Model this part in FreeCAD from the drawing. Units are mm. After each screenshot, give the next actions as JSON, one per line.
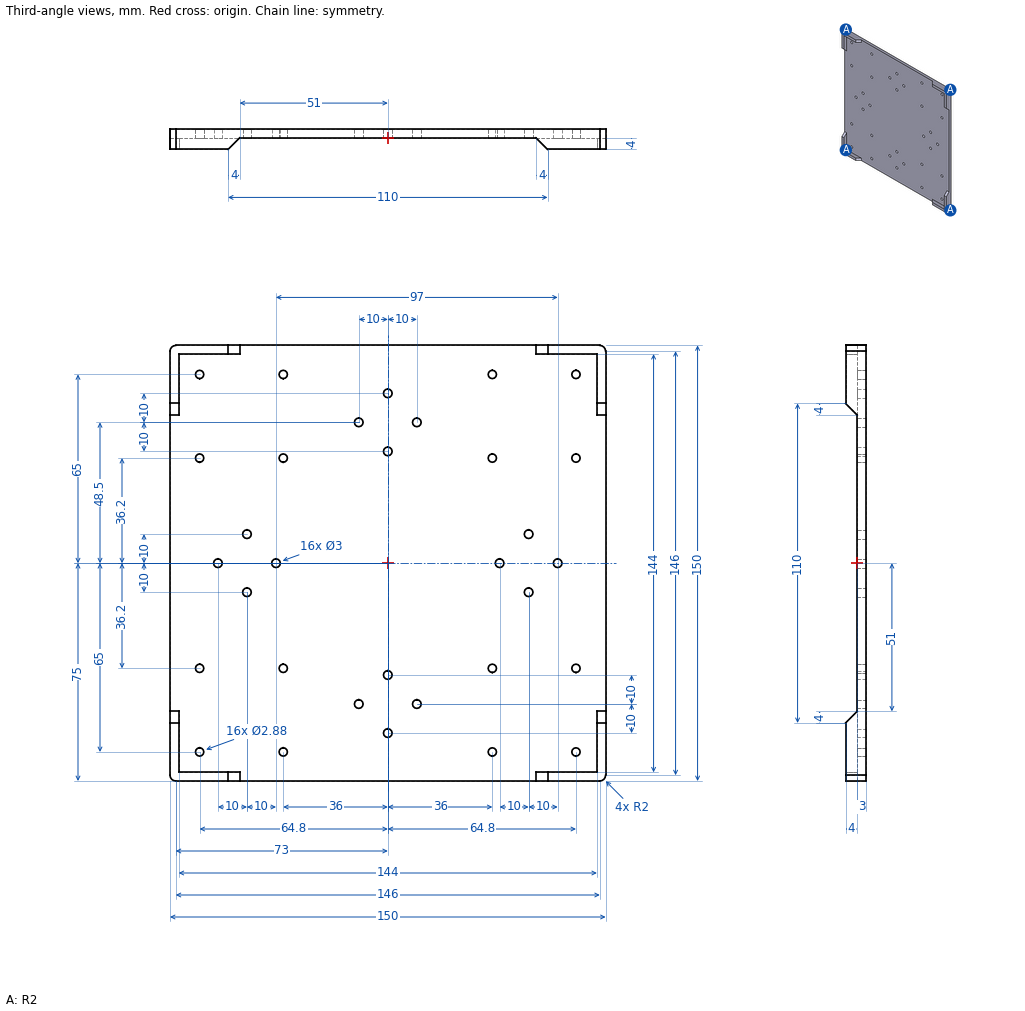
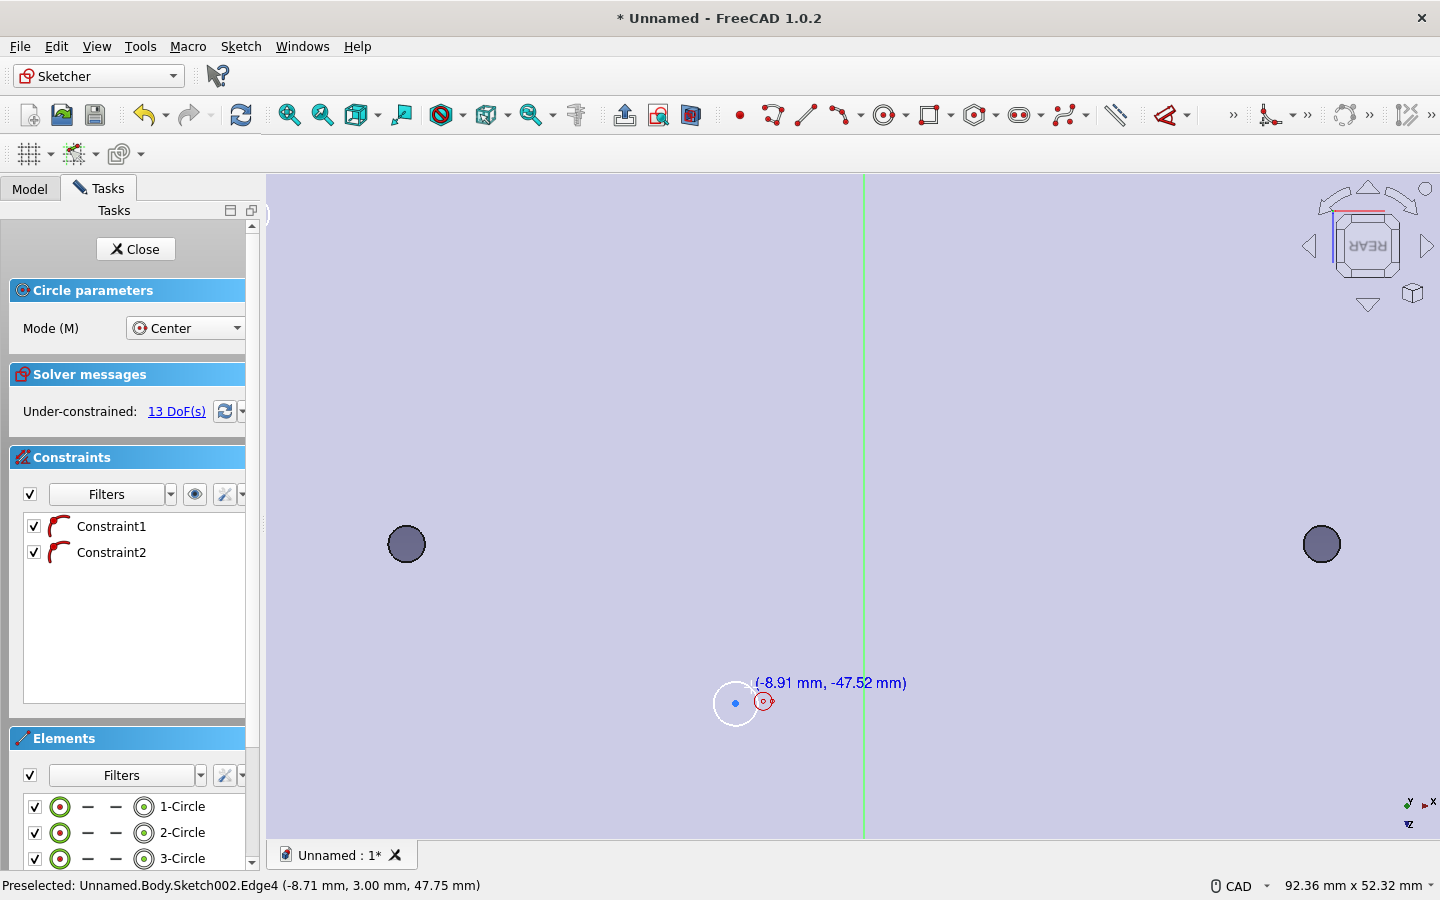
{"action": "scroll", "coordinate": [750, 689], "scroll_direction": "down", "scroll_amount": 6}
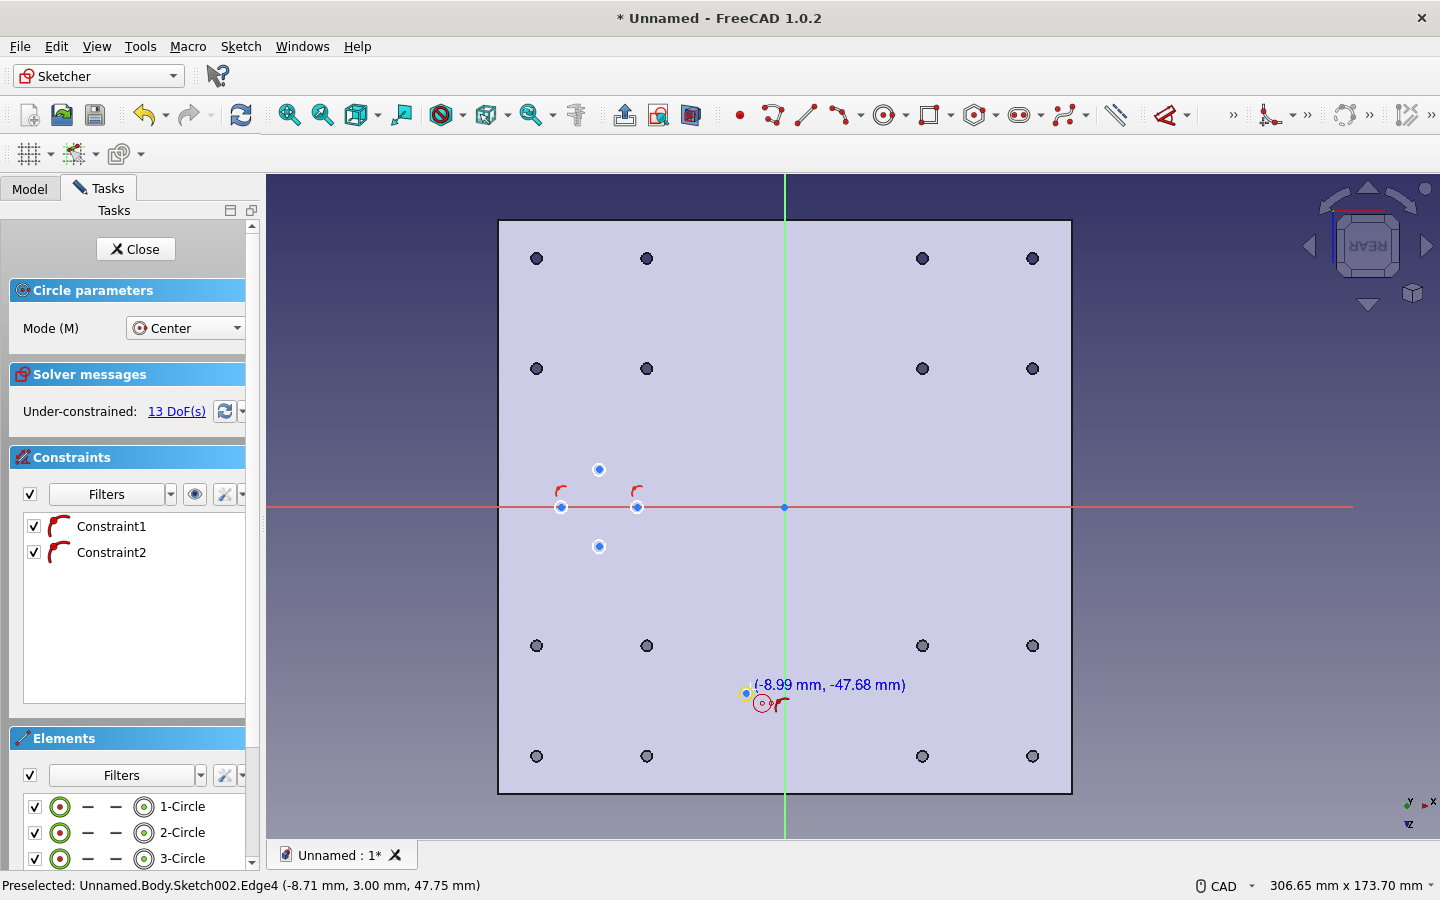
{"action": "scroll", "coordinate": [785, 731], "scroll_direction": "up", "scroll_amount": 7}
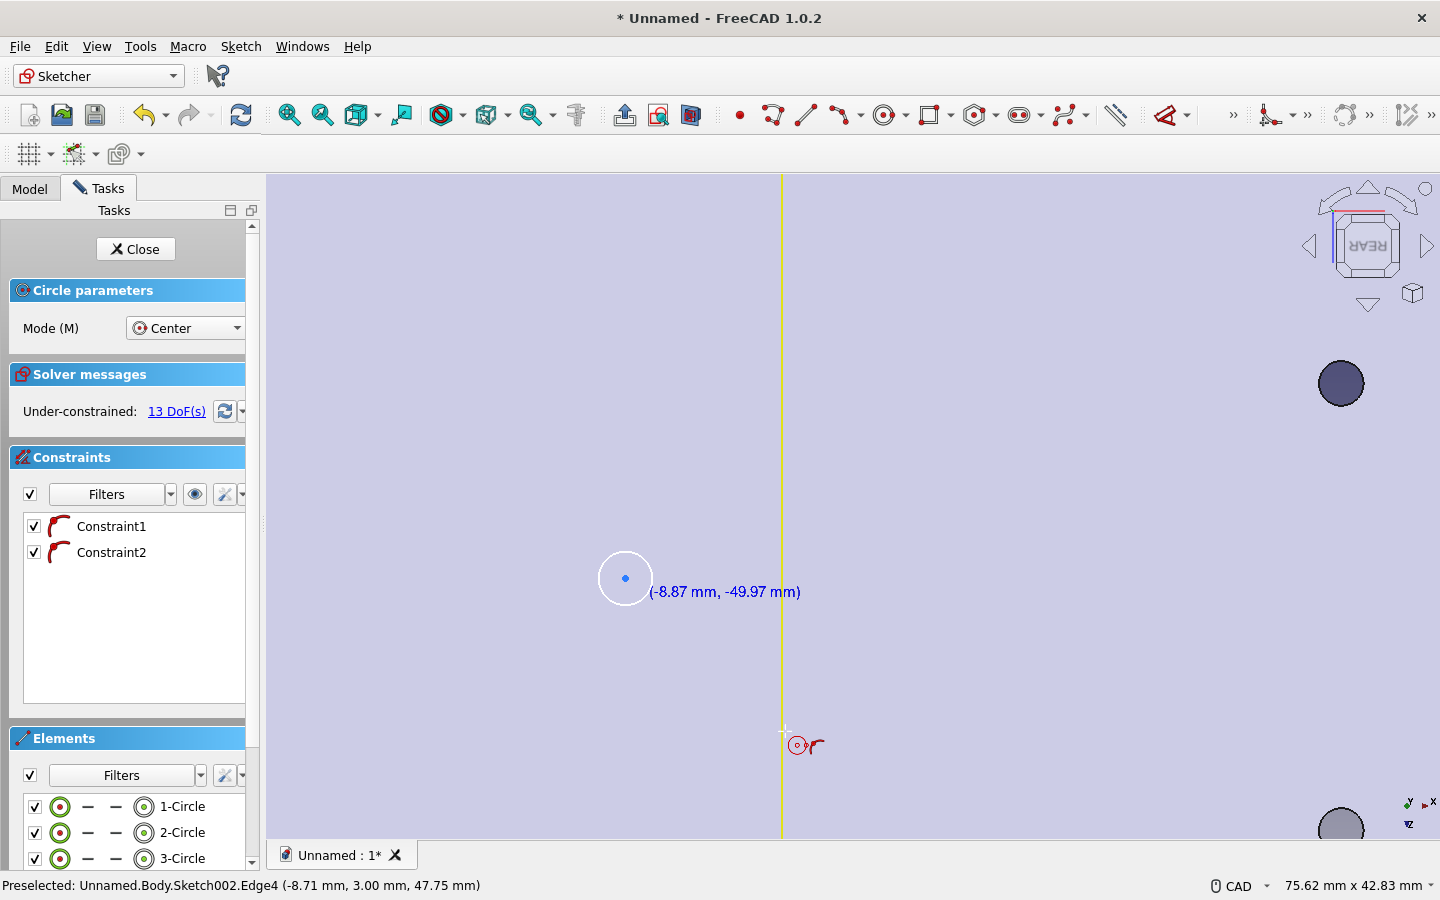
{"action": "scroll", "coordinate": [785, 731], "scroll_direction": "down", "scroll_amount": 7}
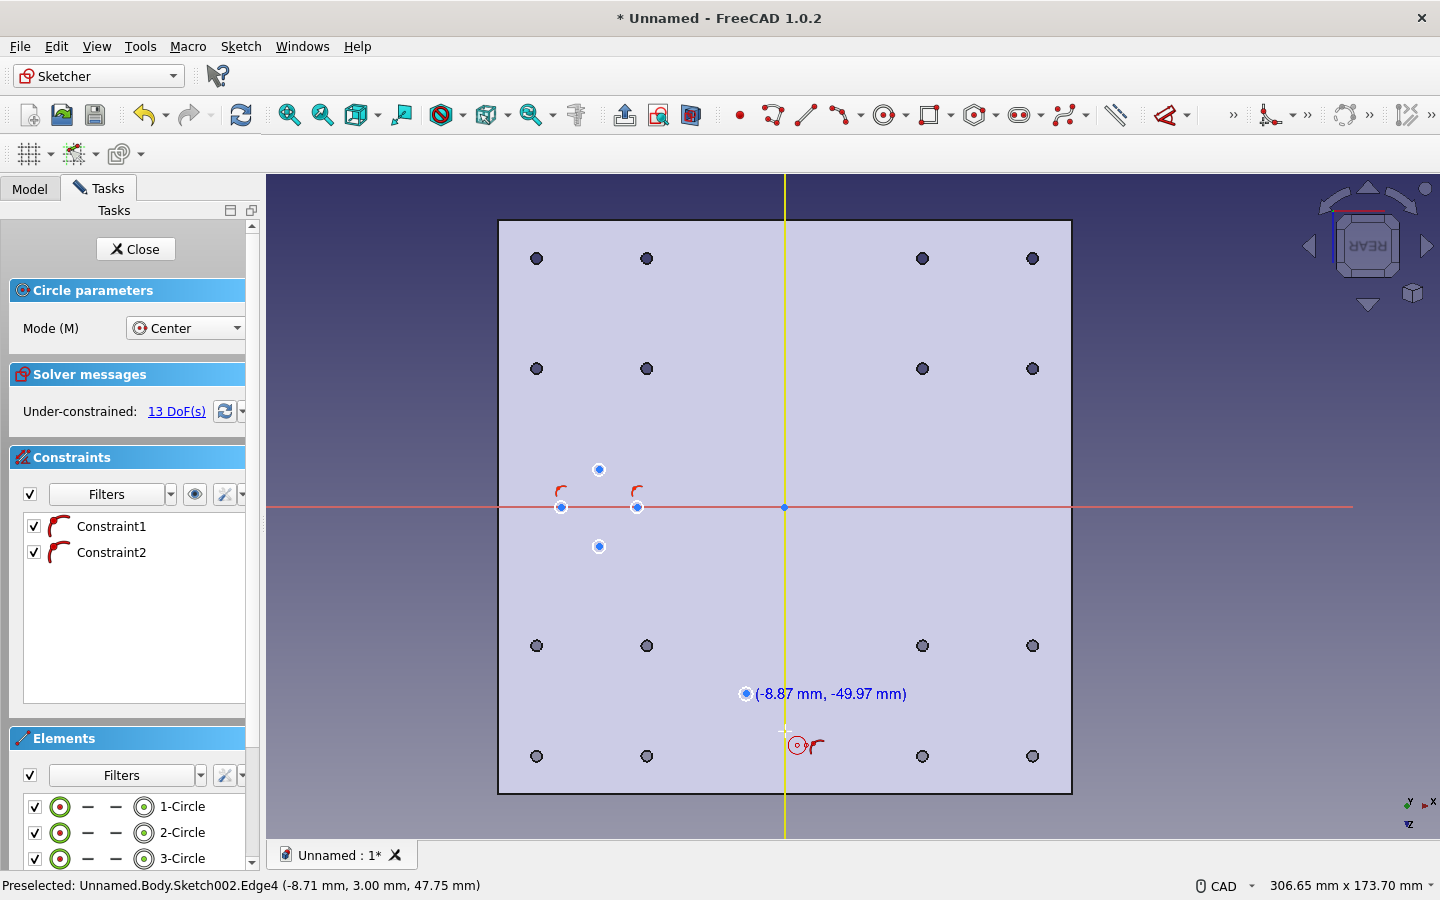
{"action": "left_click", "coordinate": [785, 731]}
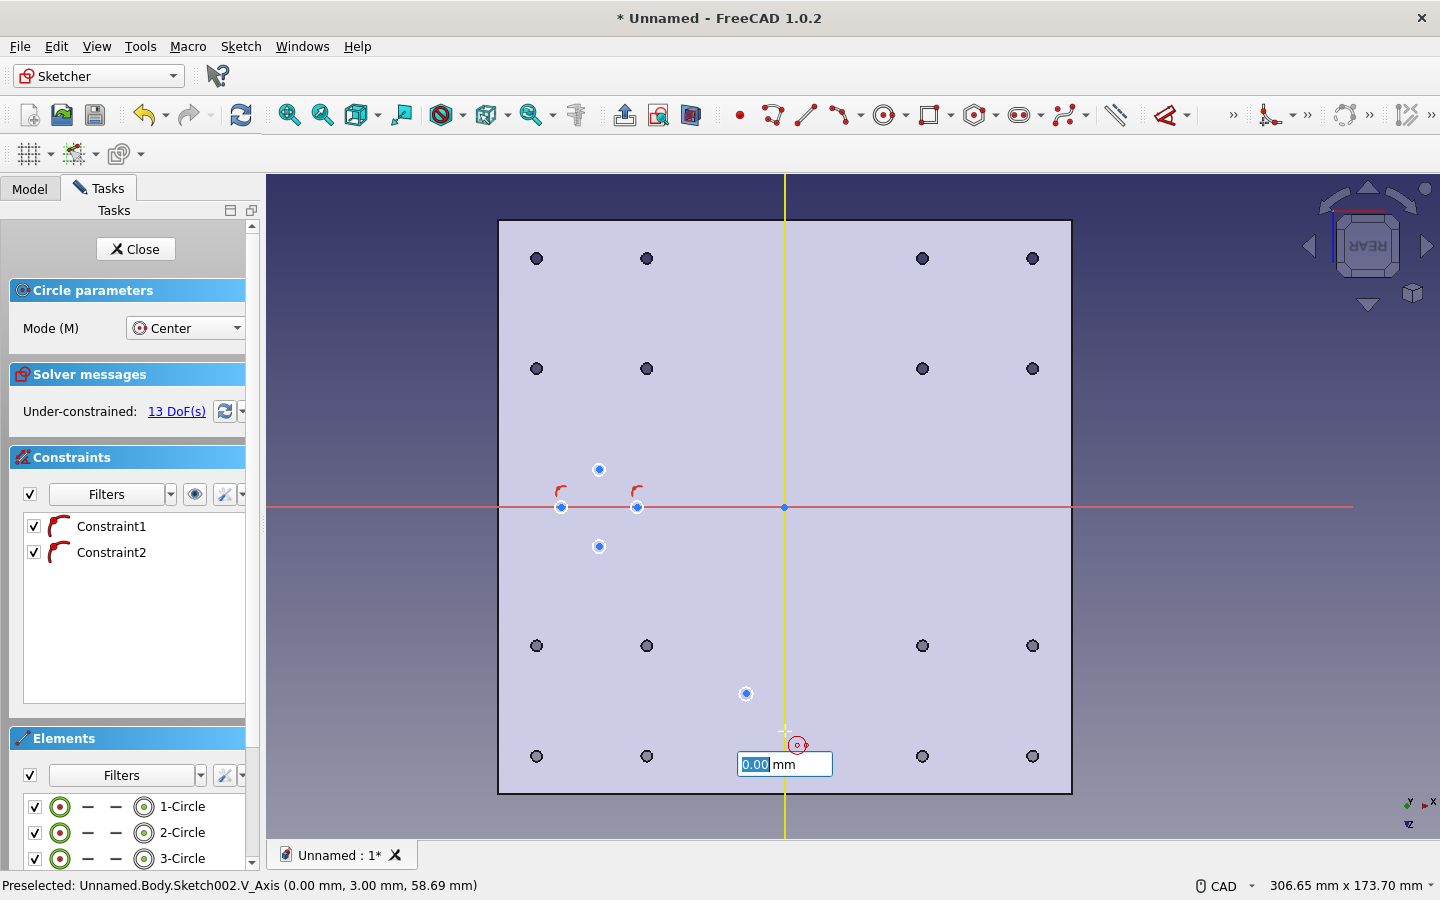
{"action": "scroll", "coordinate": [790, 729], "scroll_direction": "up", "scroll_amount": 6}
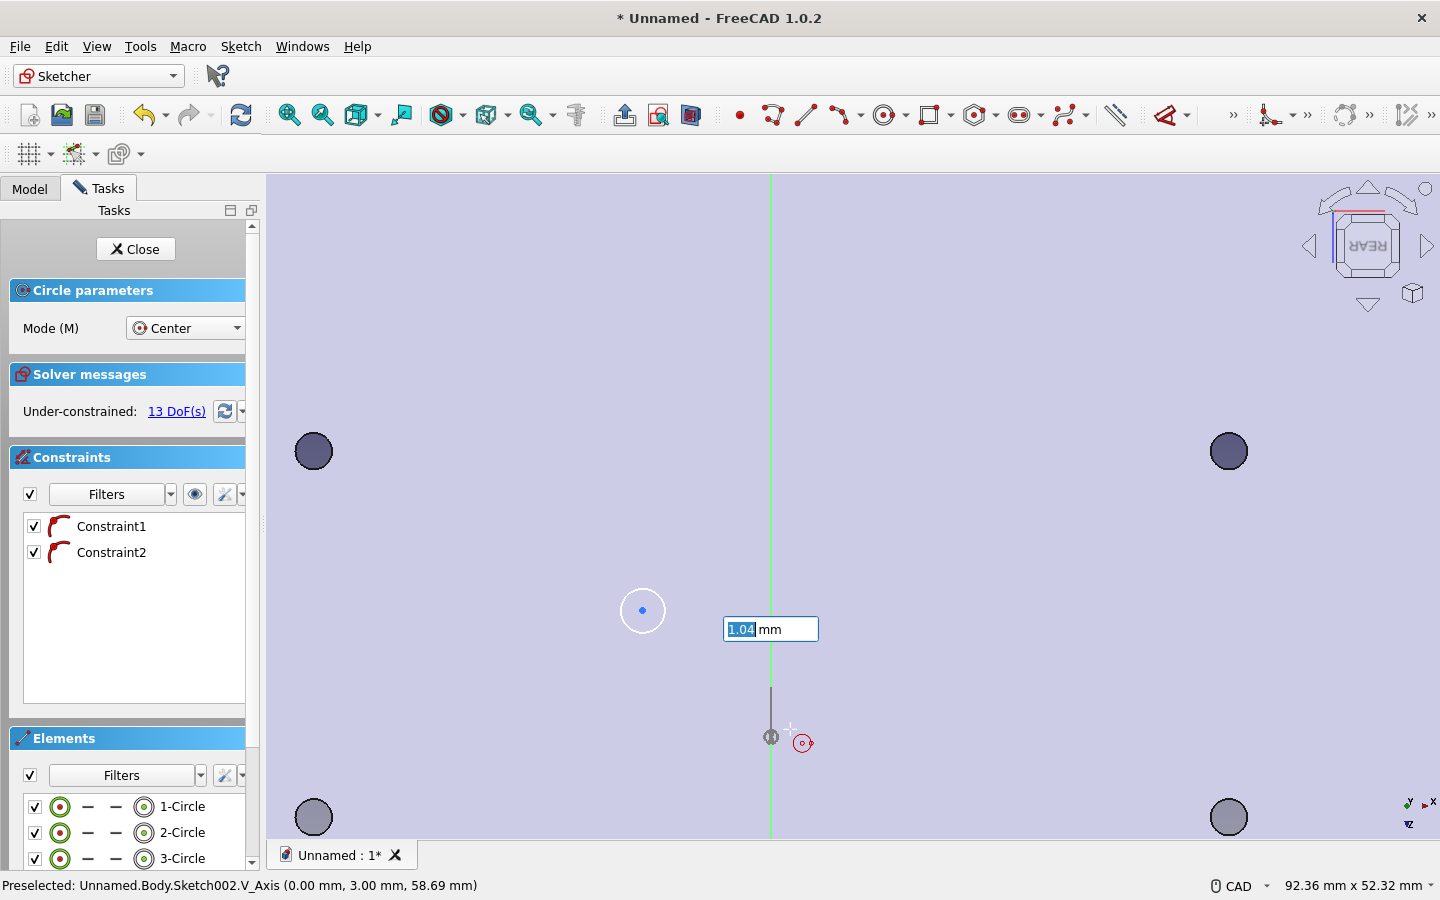
{"action": "left_click", "coordinate": [789, 728]}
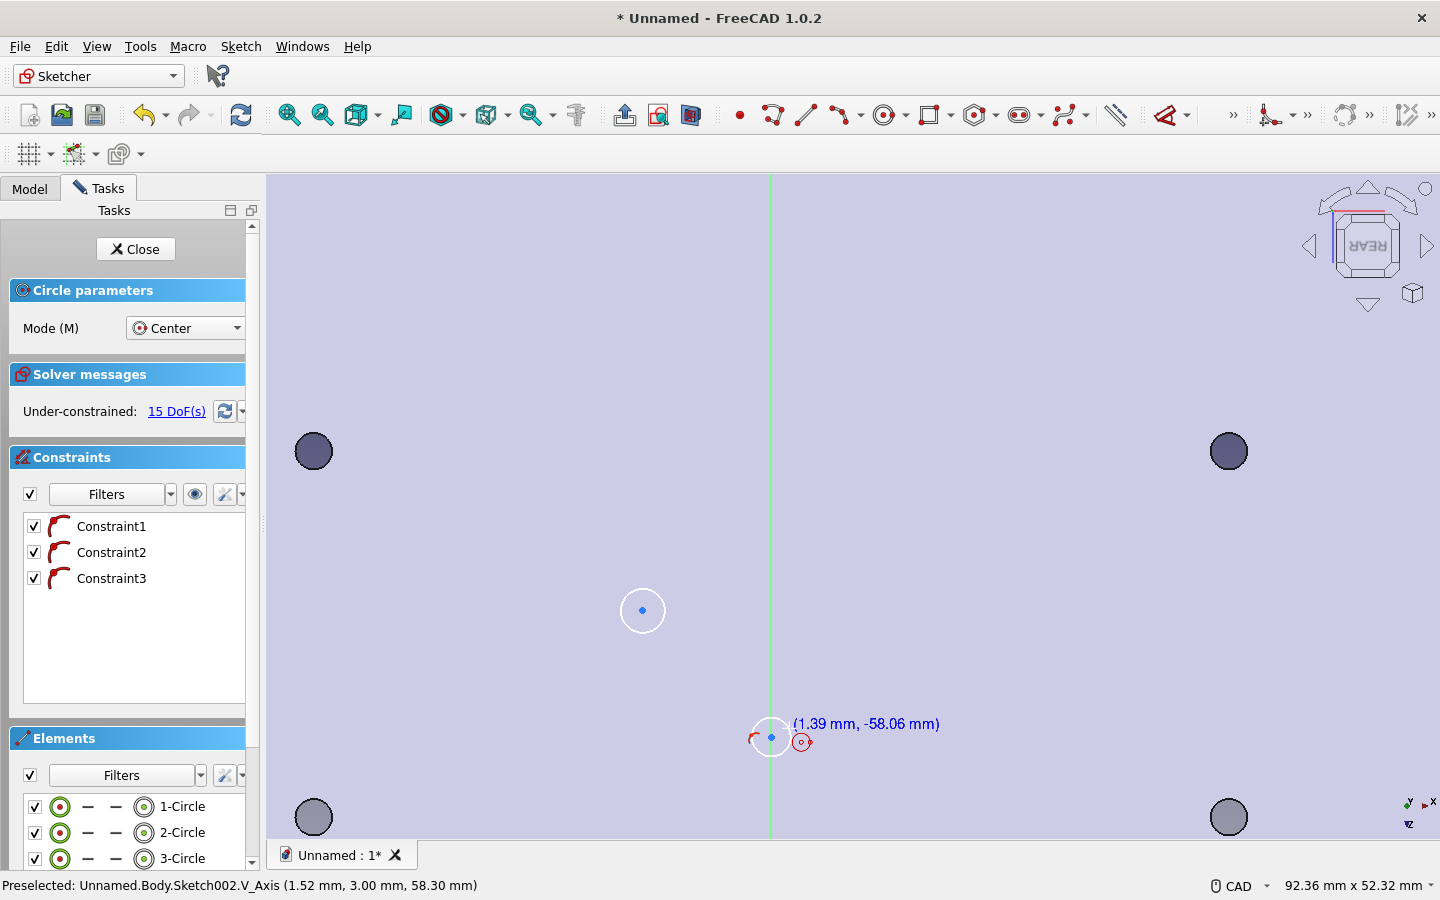
{"action": "scroll", "coordinate": [790, 729], "scroll_direction": "down", "scroll_amount": 6}